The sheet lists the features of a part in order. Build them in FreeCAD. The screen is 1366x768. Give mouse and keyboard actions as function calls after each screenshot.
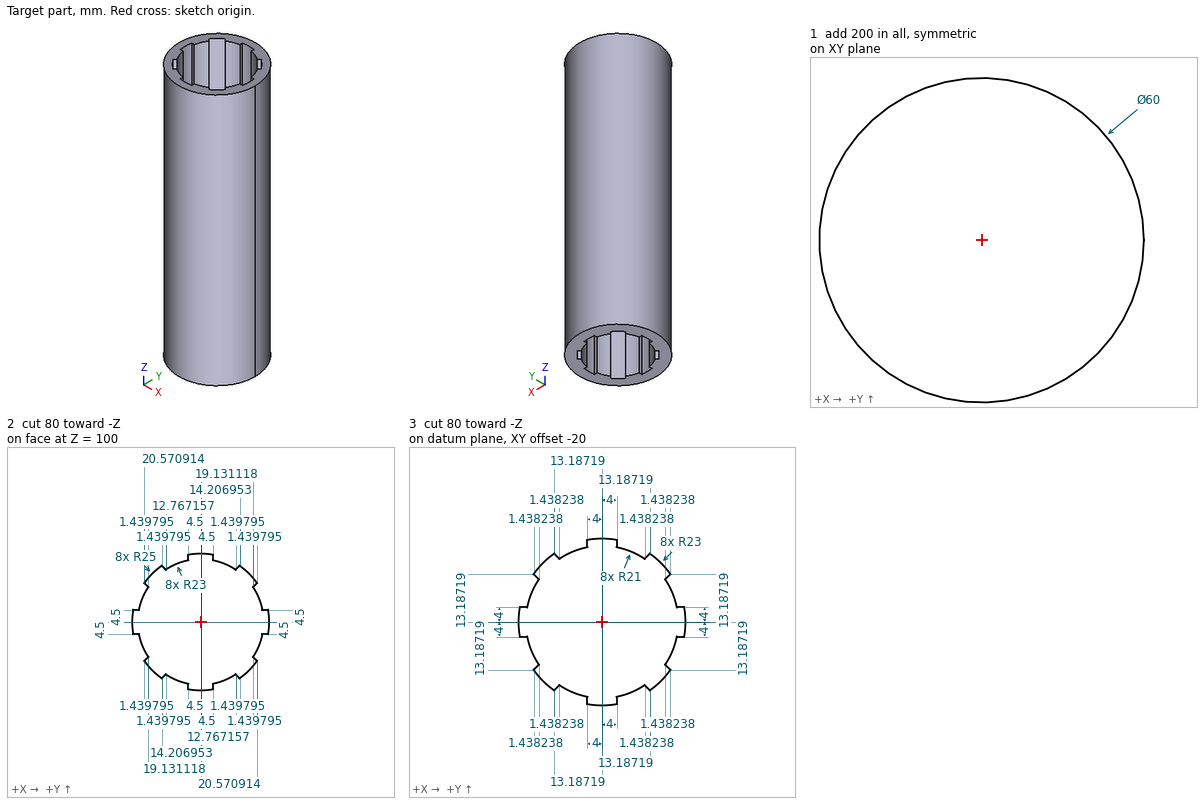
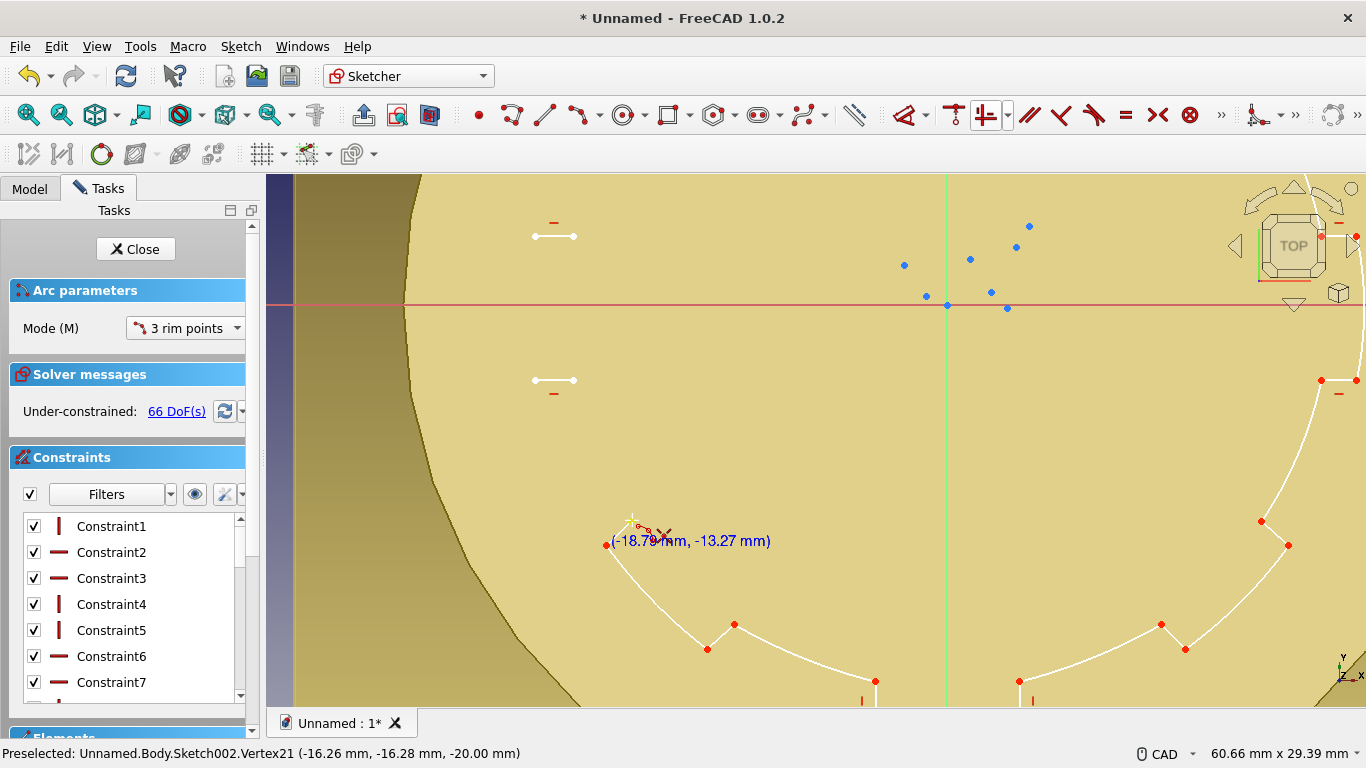
click(631, 521)
click(574, 380)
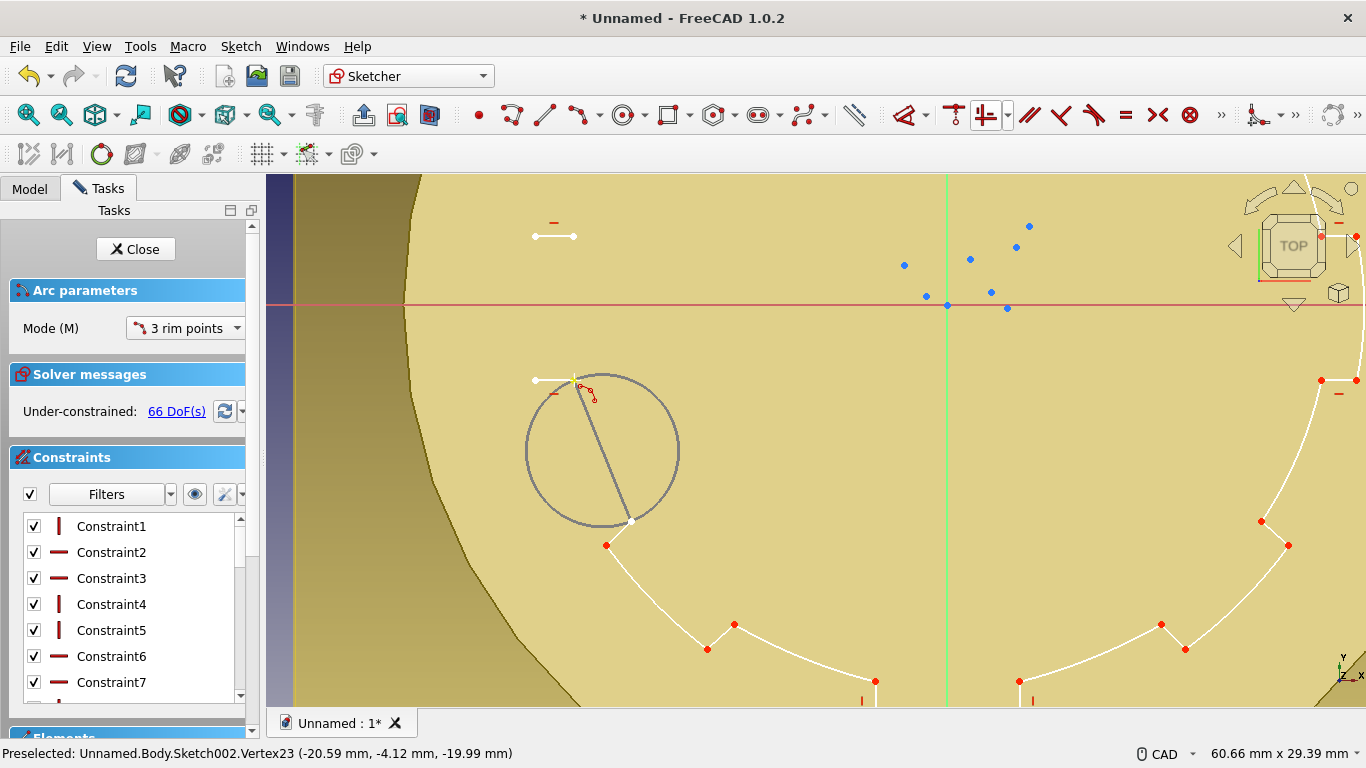
scroll(596, 451, up, 4)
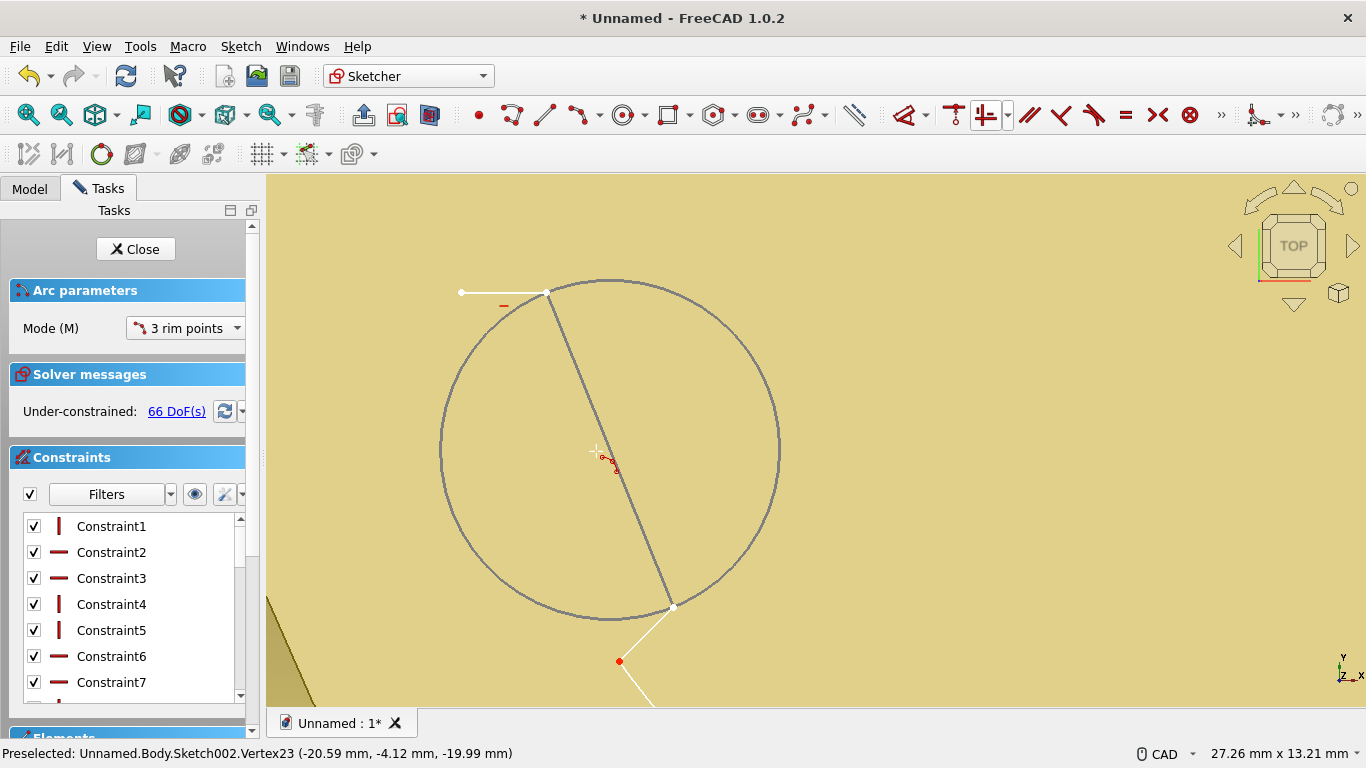
click(595, 450)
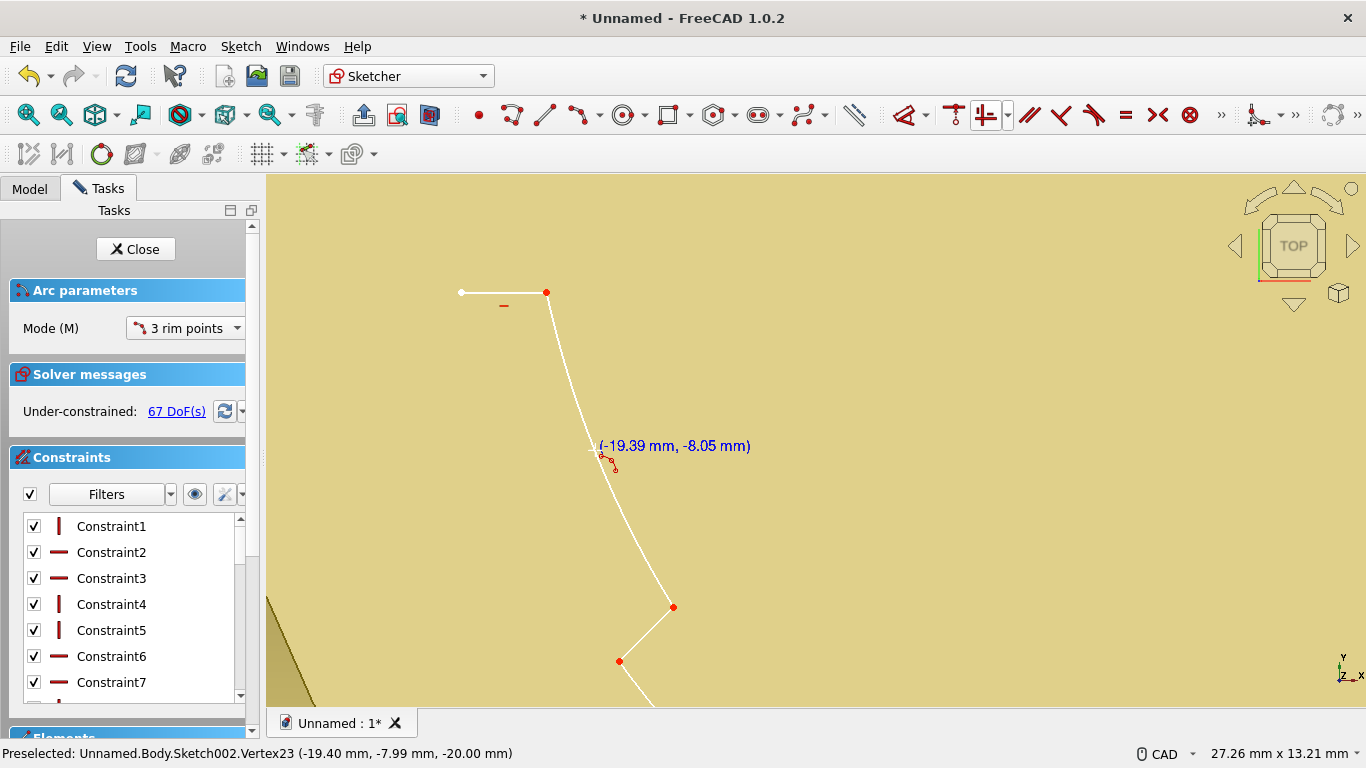
click(462, 293)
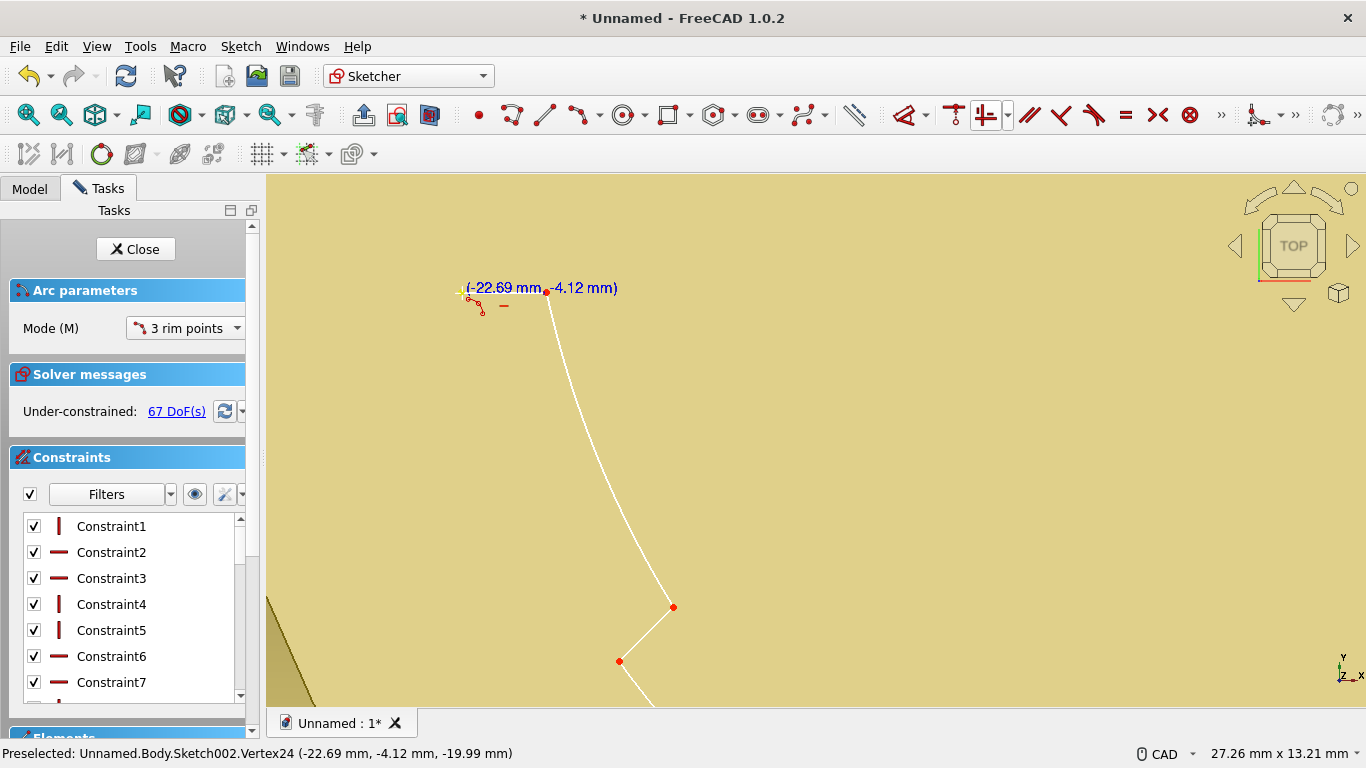
scroll(623, 503, down, 9)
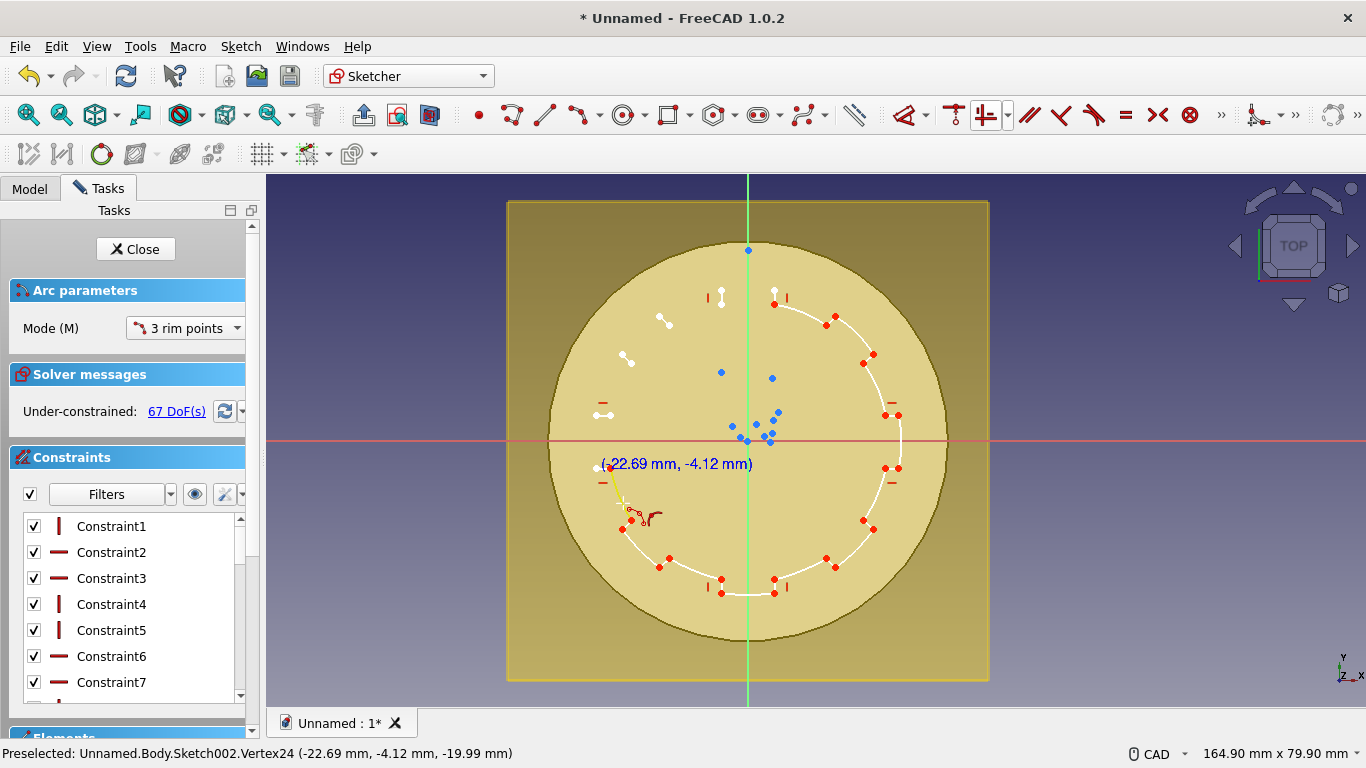
scroll(597, 415, up, 5)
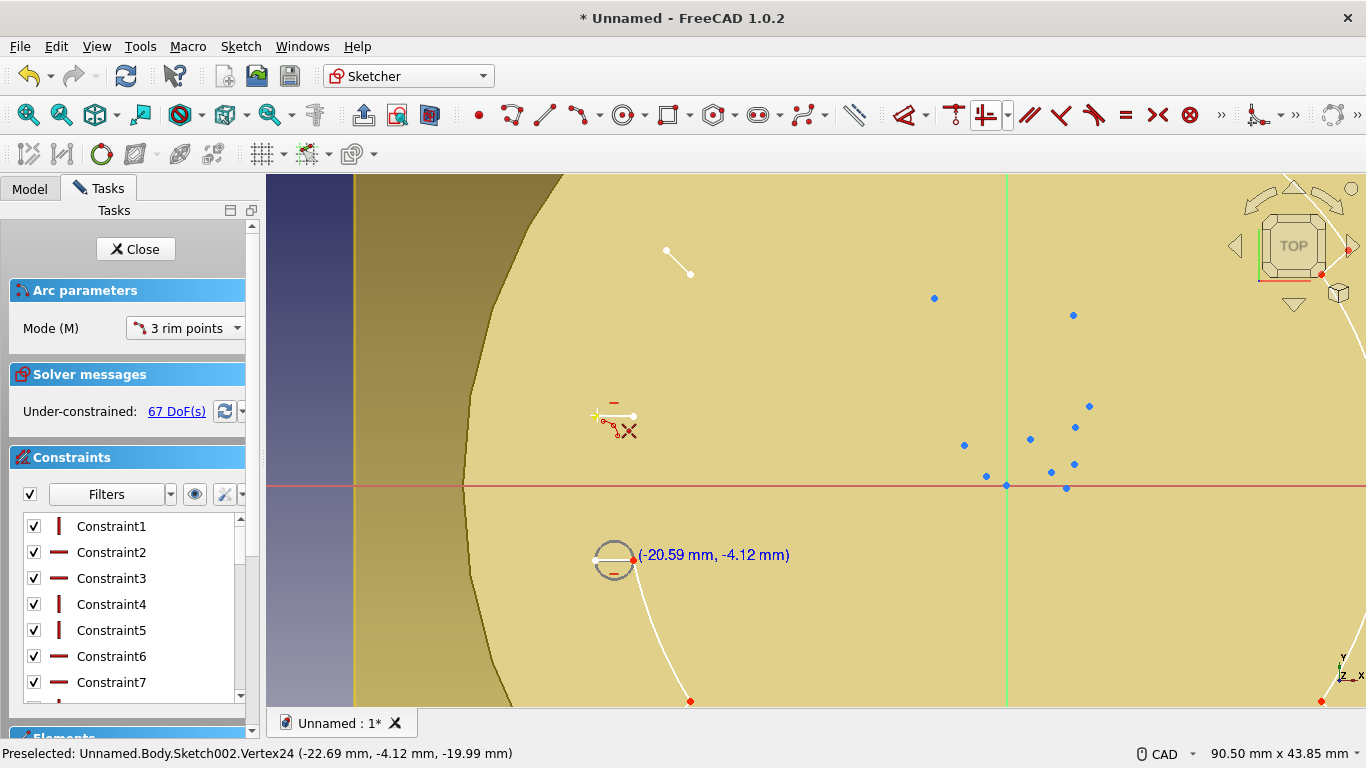
click(596, 416)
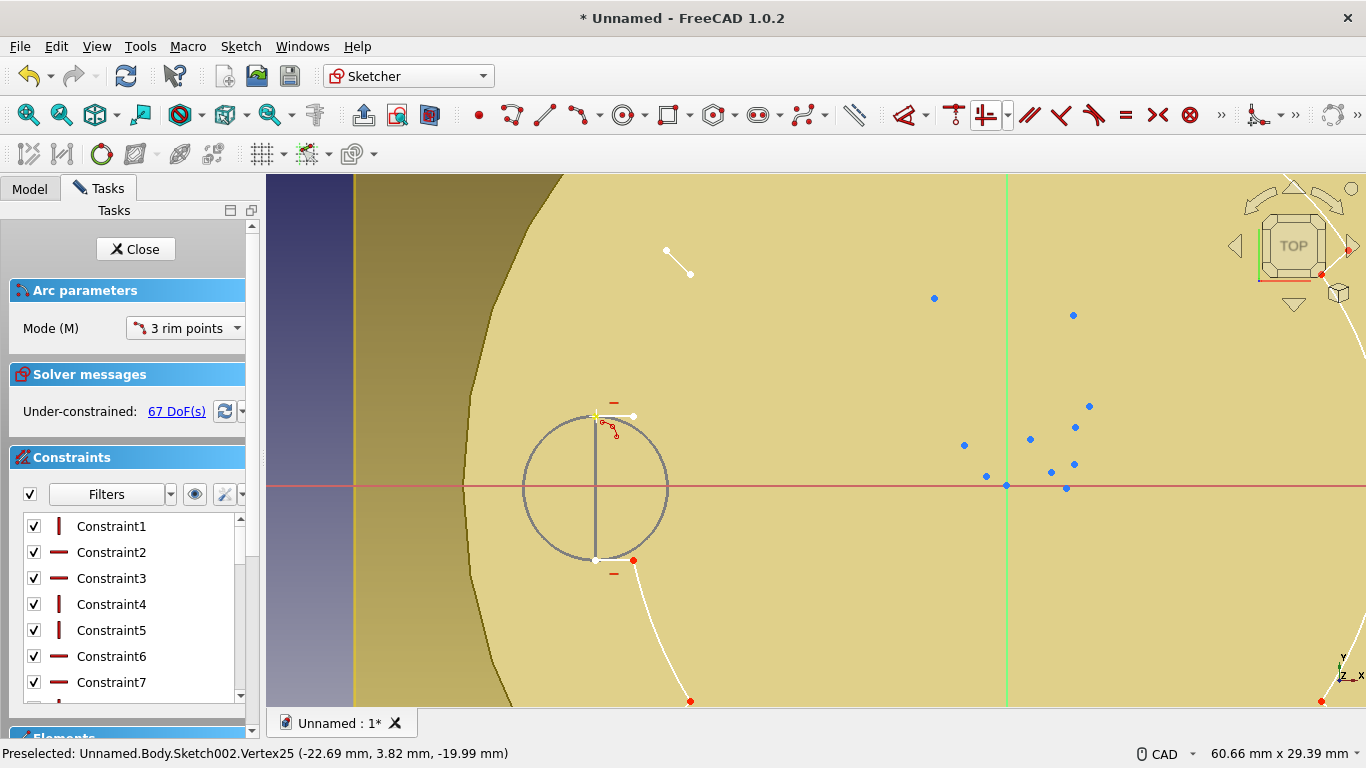
scroll(590, 471, up, 5)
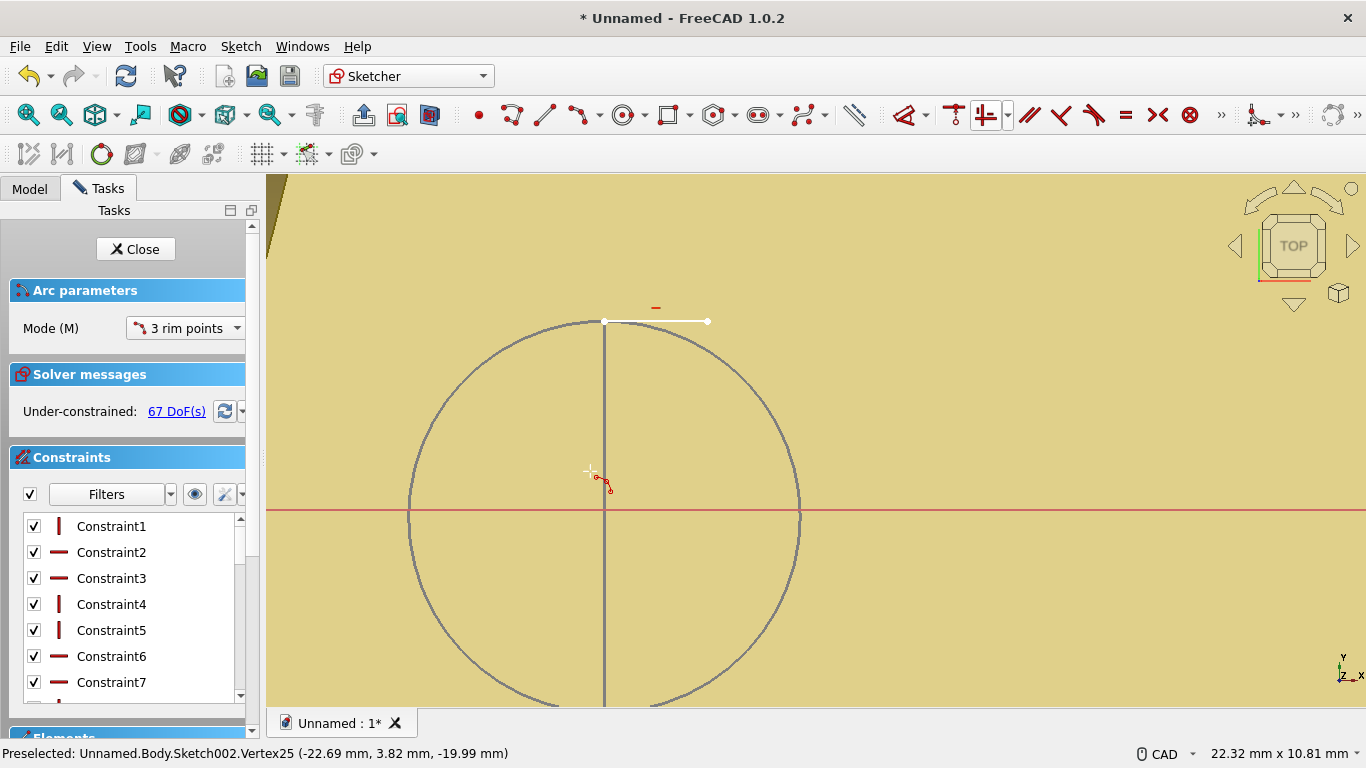
click(590, 470)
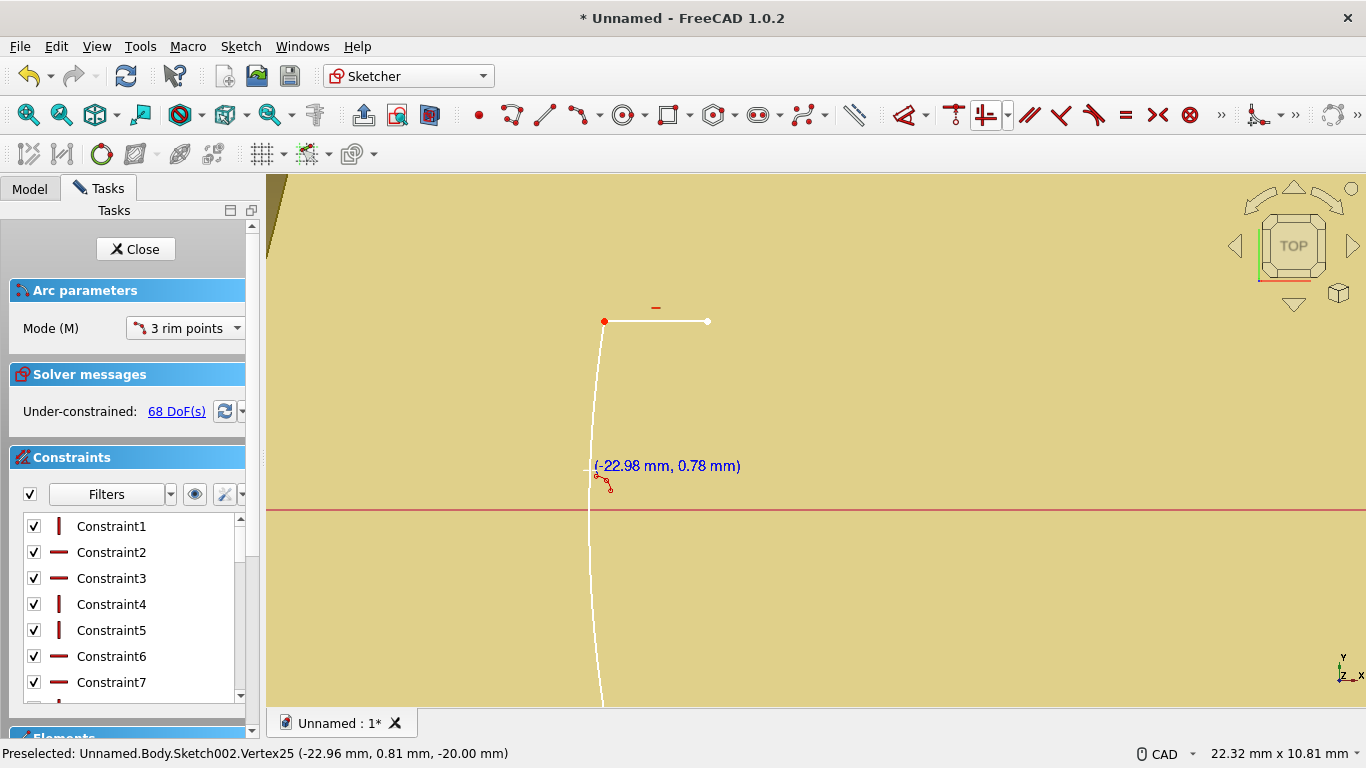
scroll(595, 430, down, 10)